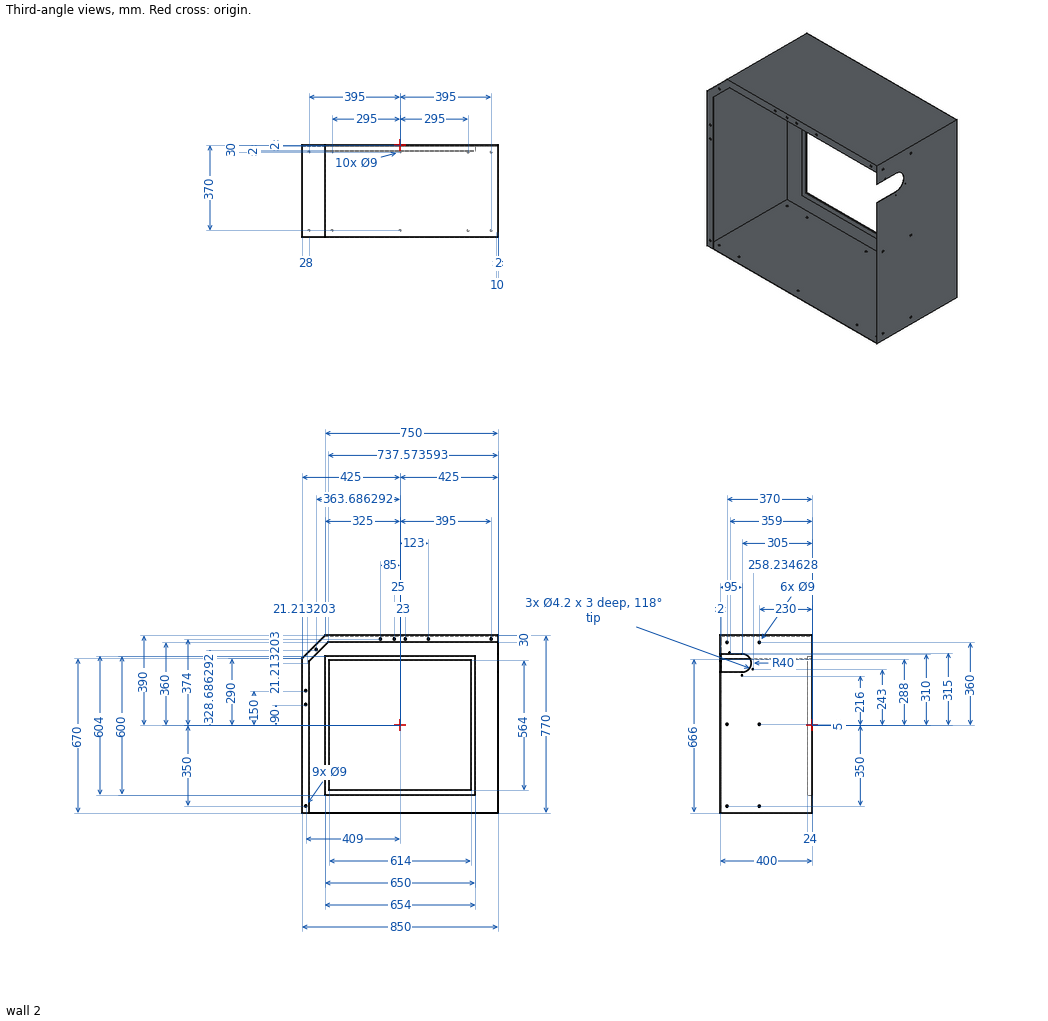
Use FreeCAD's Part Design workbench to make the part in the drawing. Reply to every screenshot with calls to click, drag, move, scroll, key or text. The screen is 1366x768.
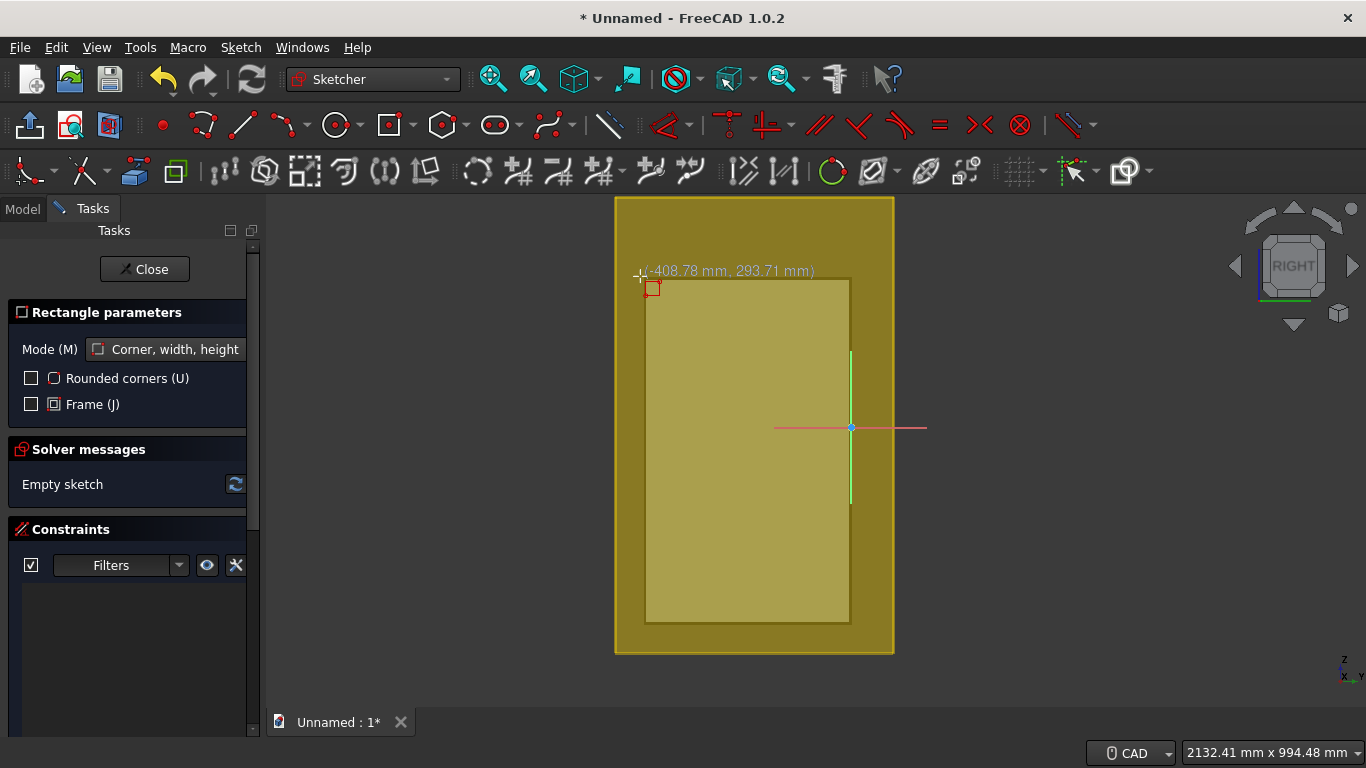
click(645, 279)
move(646, 623)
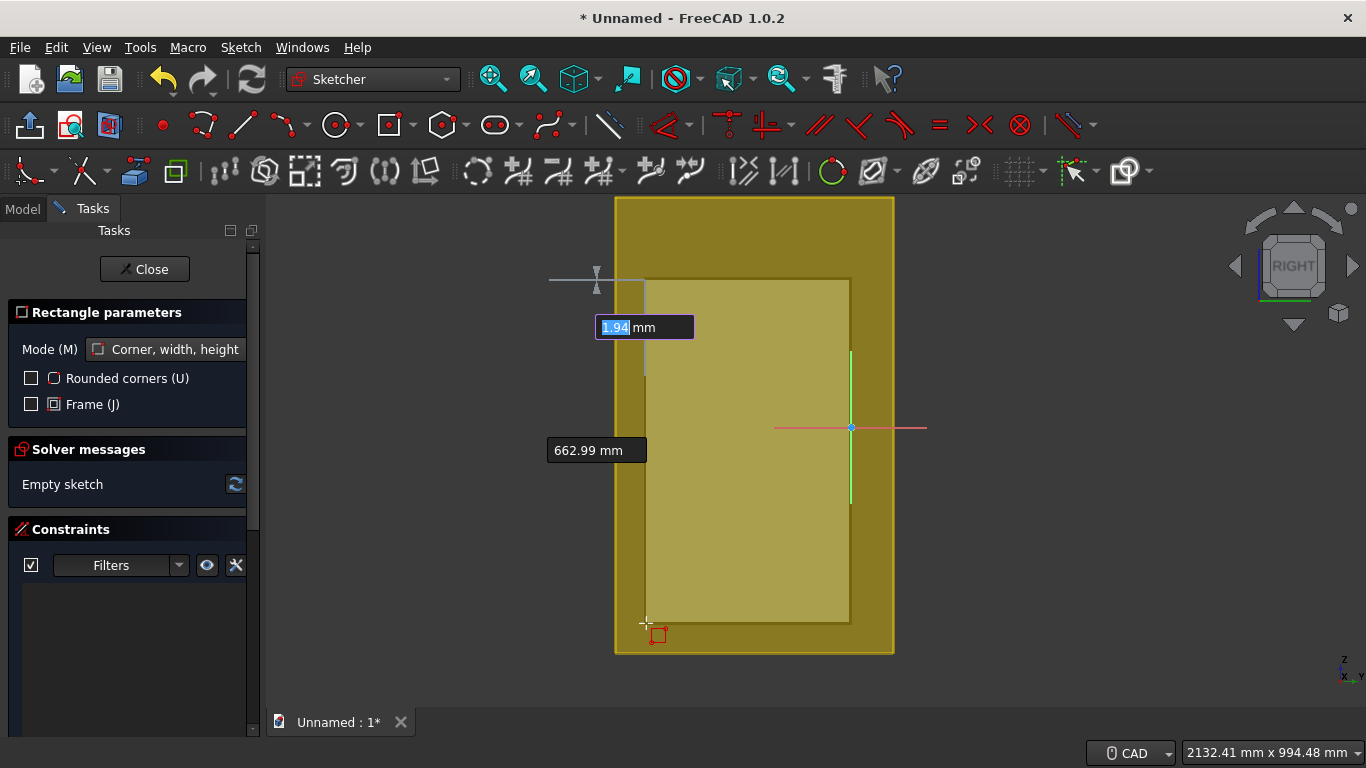
text(2)
key(Tab)
text(666)
key(Return)
key(Escape)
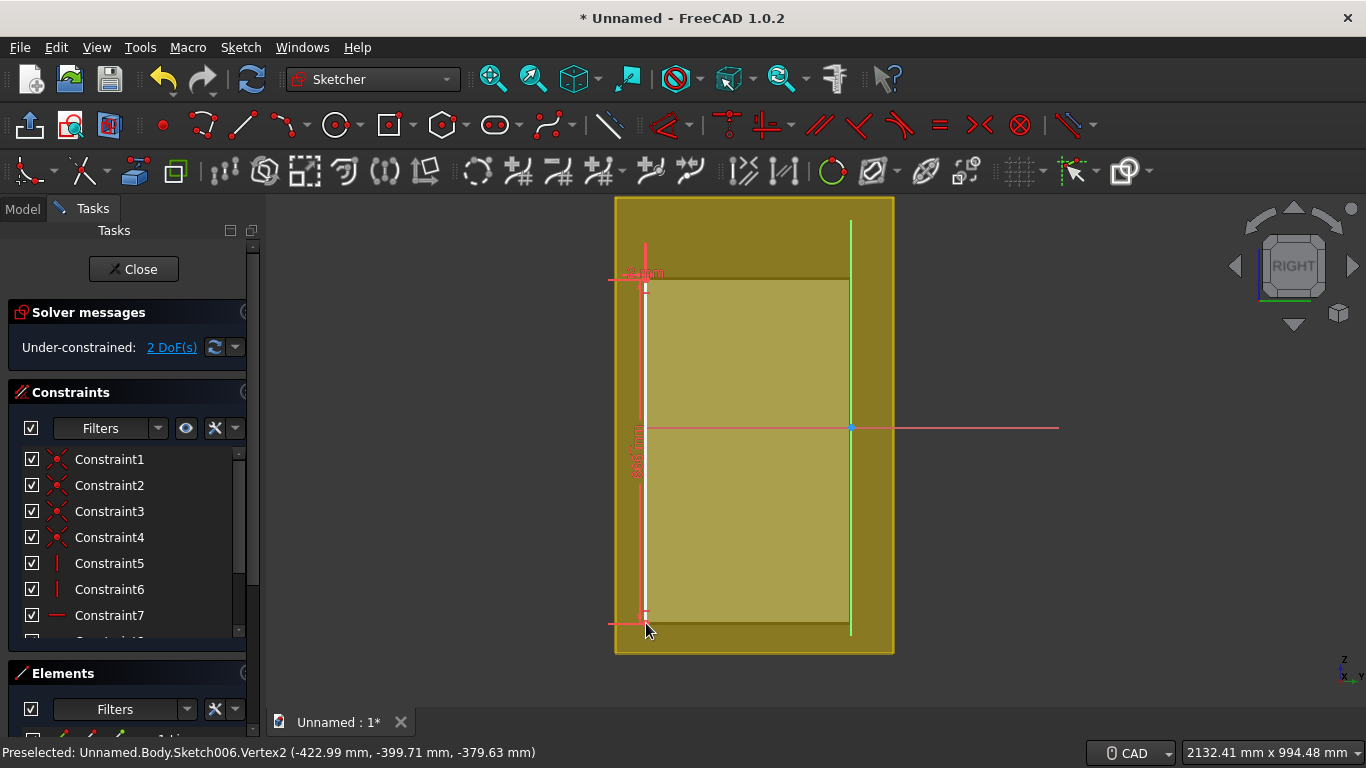
click(664, 126)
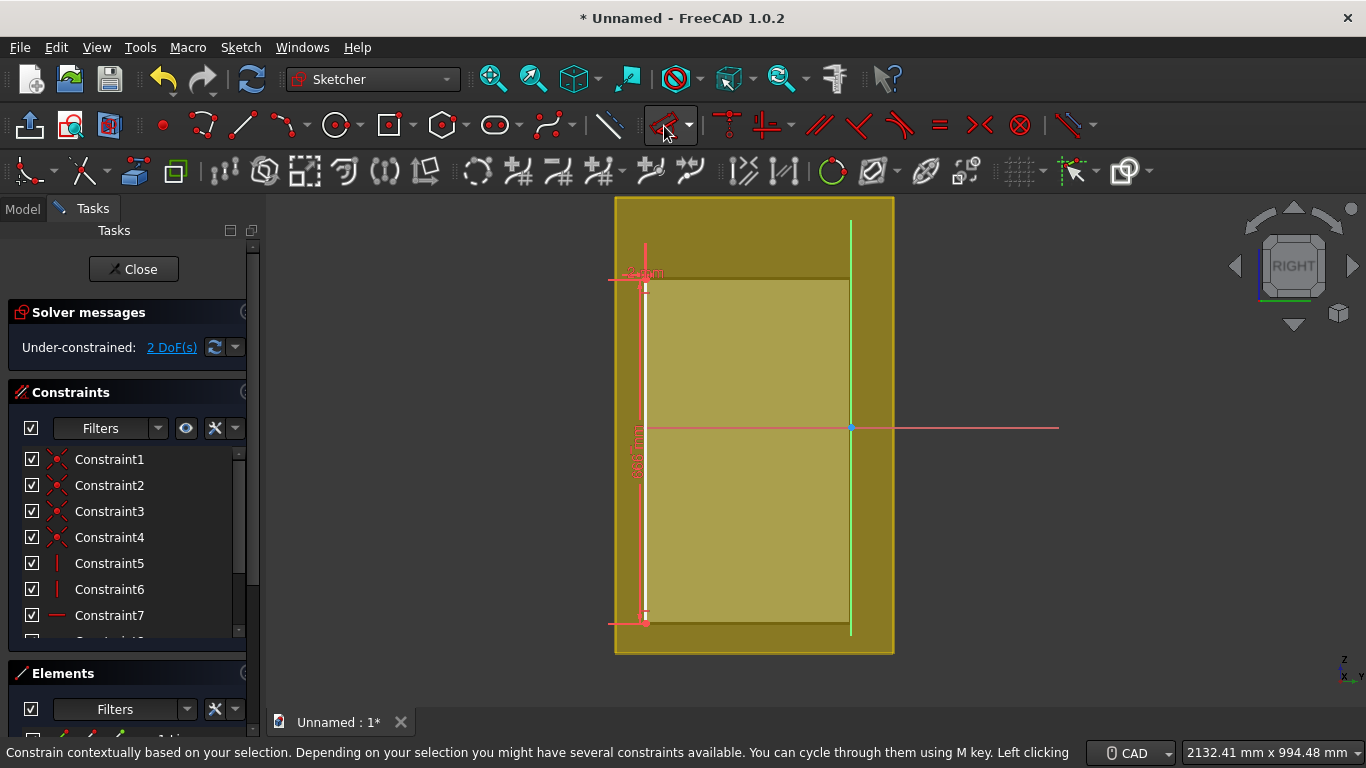
scroll(645, 280, up, 13)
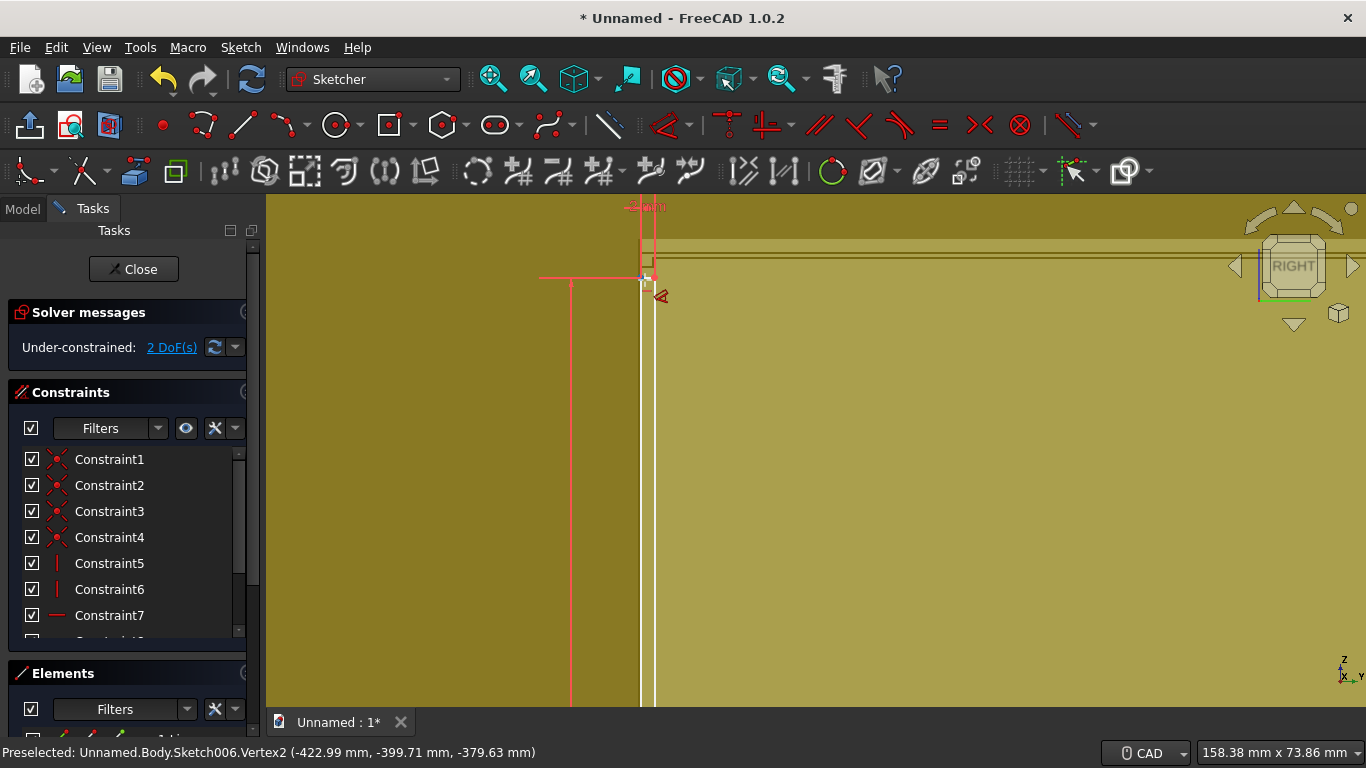
click(641, 278)
click(921, 244)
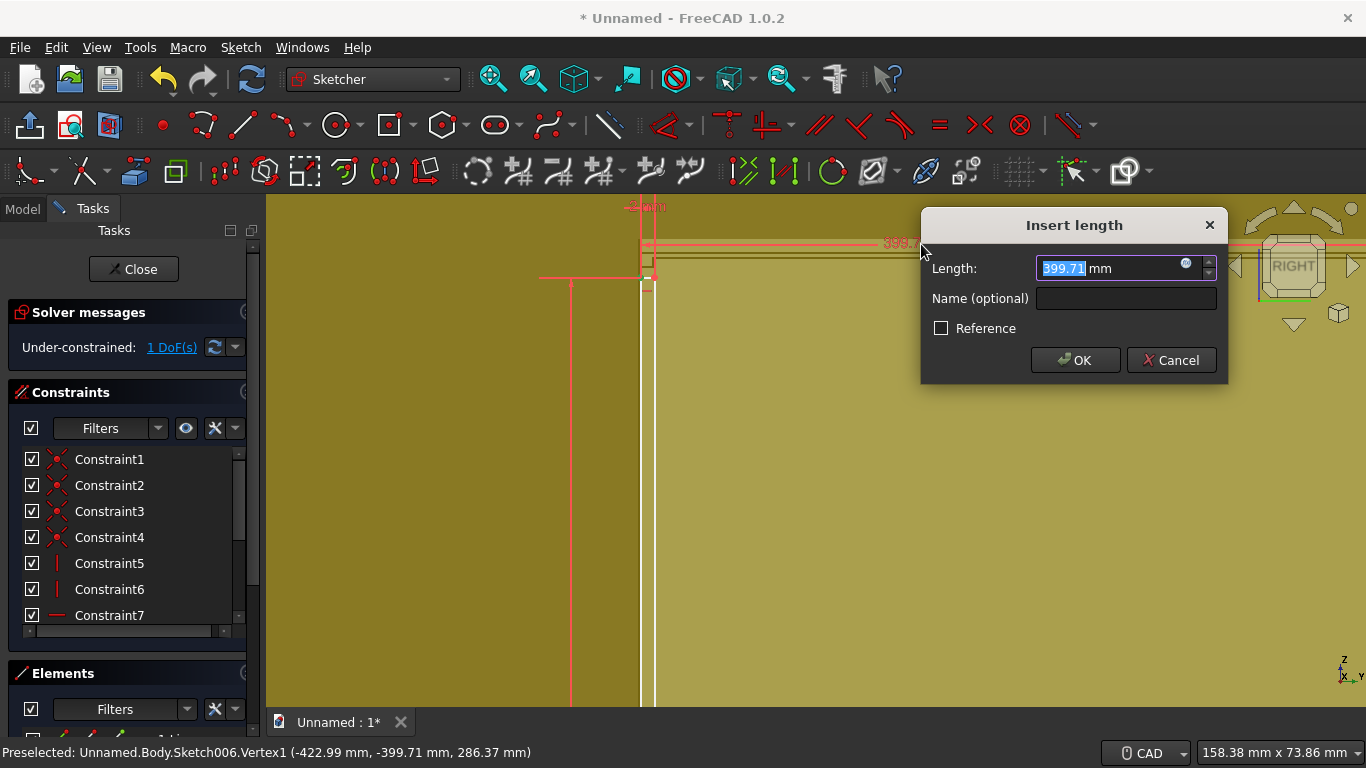
text(400)
key(Return)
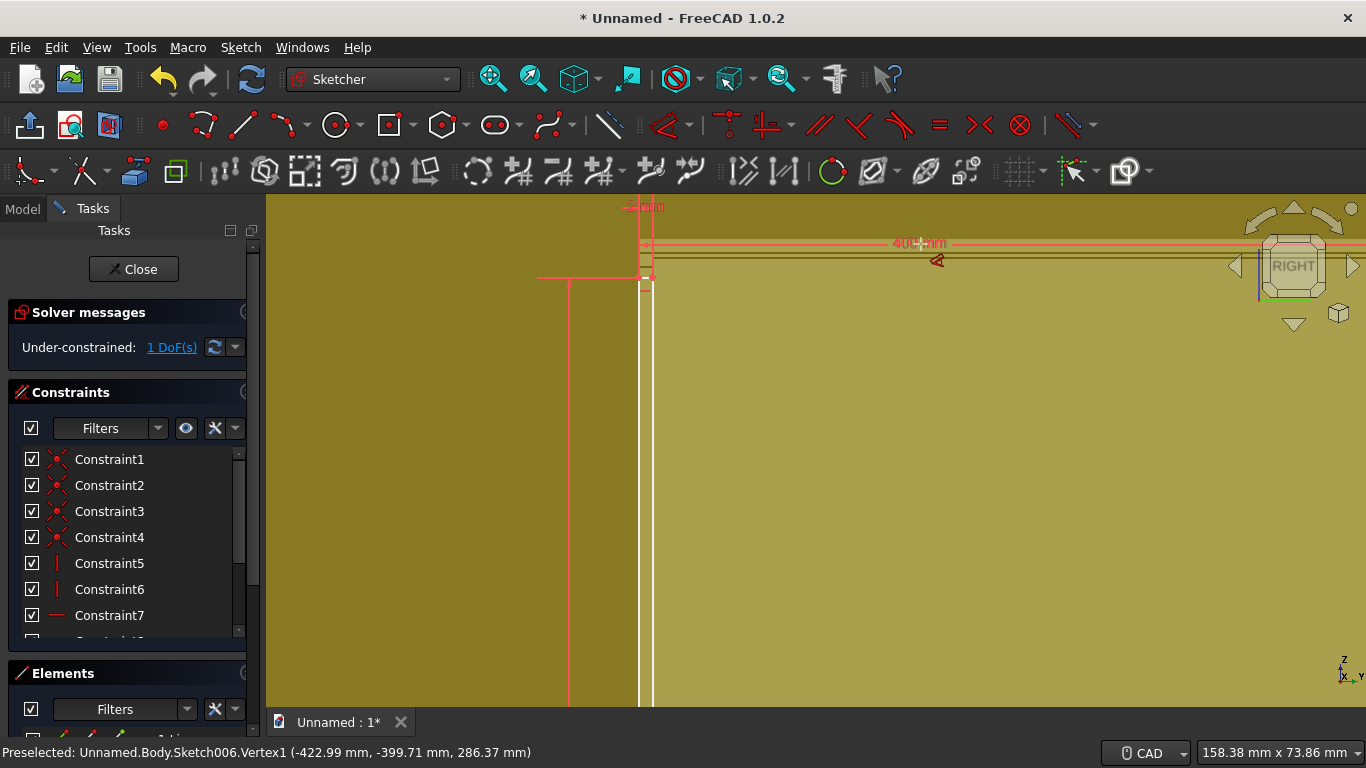
click(639, 278)
click(605, 478)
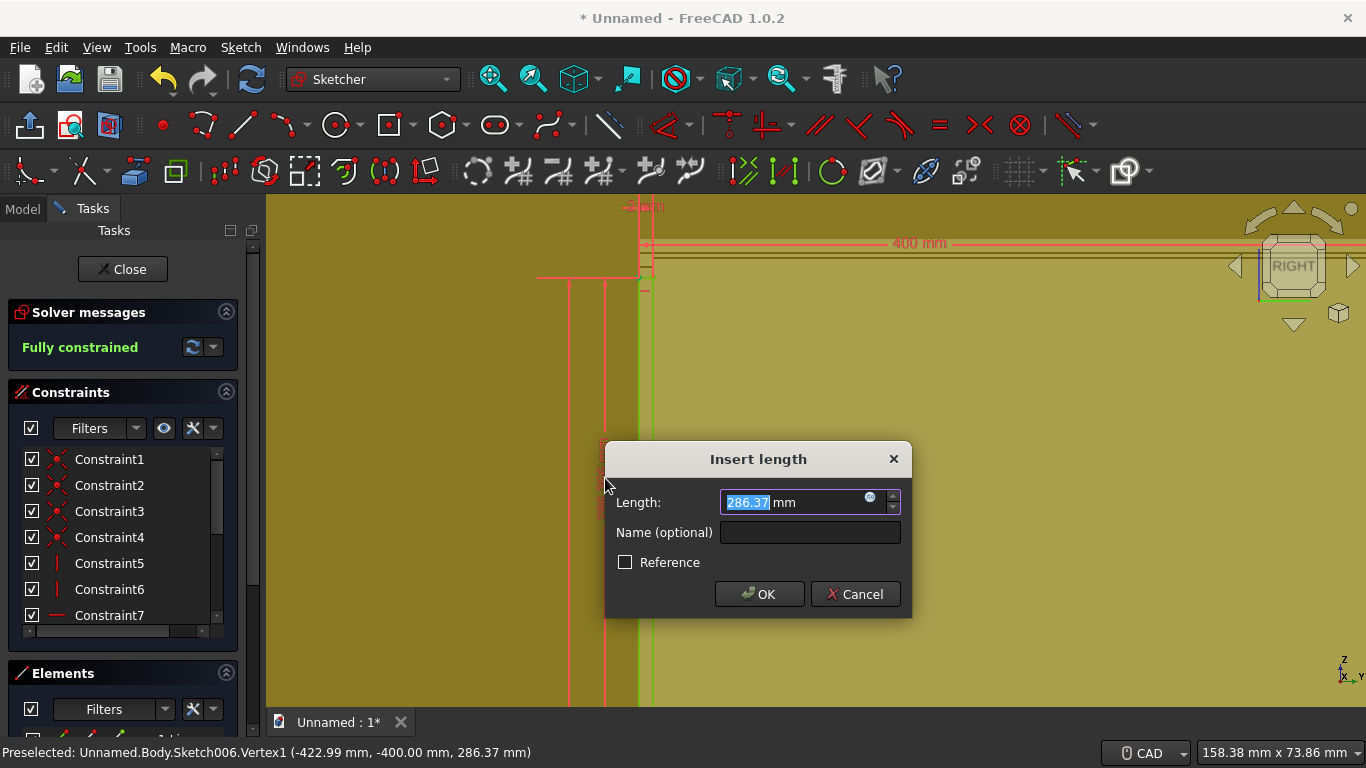
text(288)
key(Return)
key(Escape)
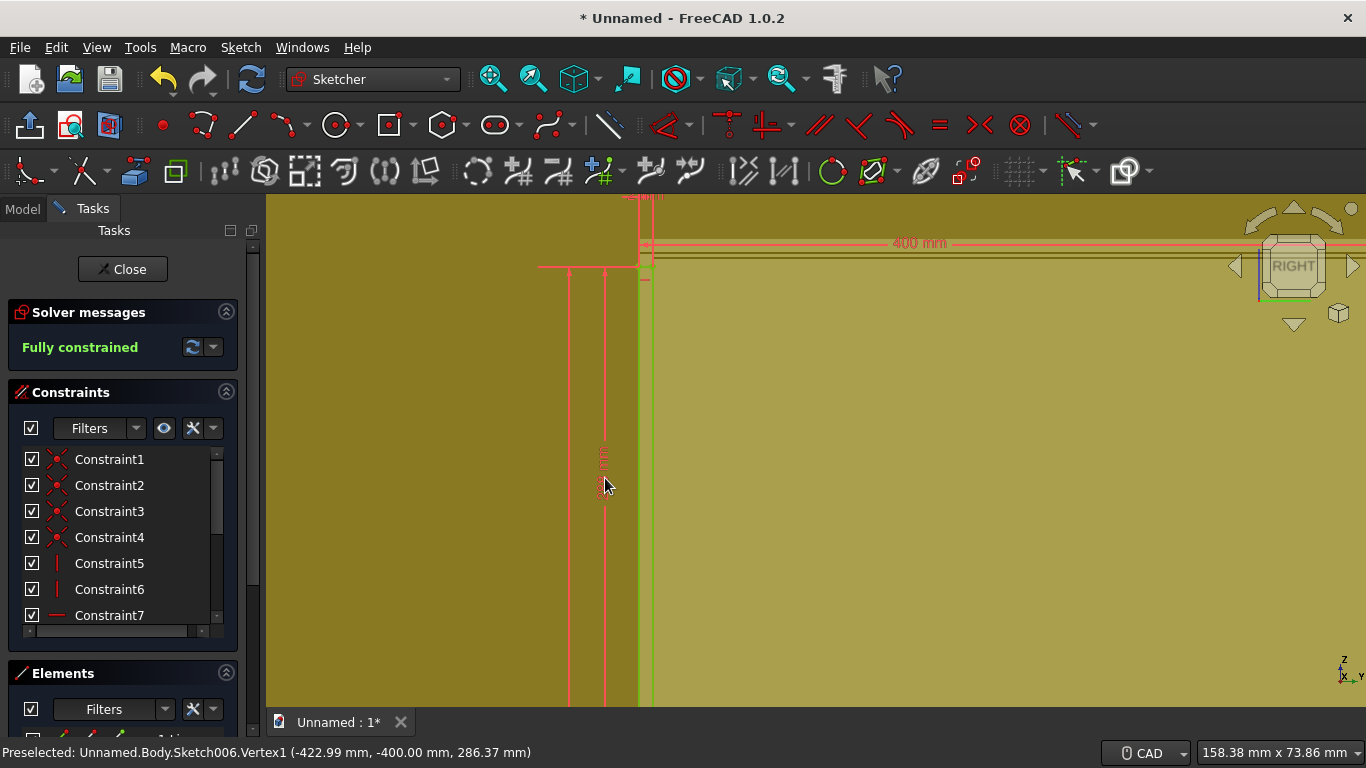
click(123, 269)